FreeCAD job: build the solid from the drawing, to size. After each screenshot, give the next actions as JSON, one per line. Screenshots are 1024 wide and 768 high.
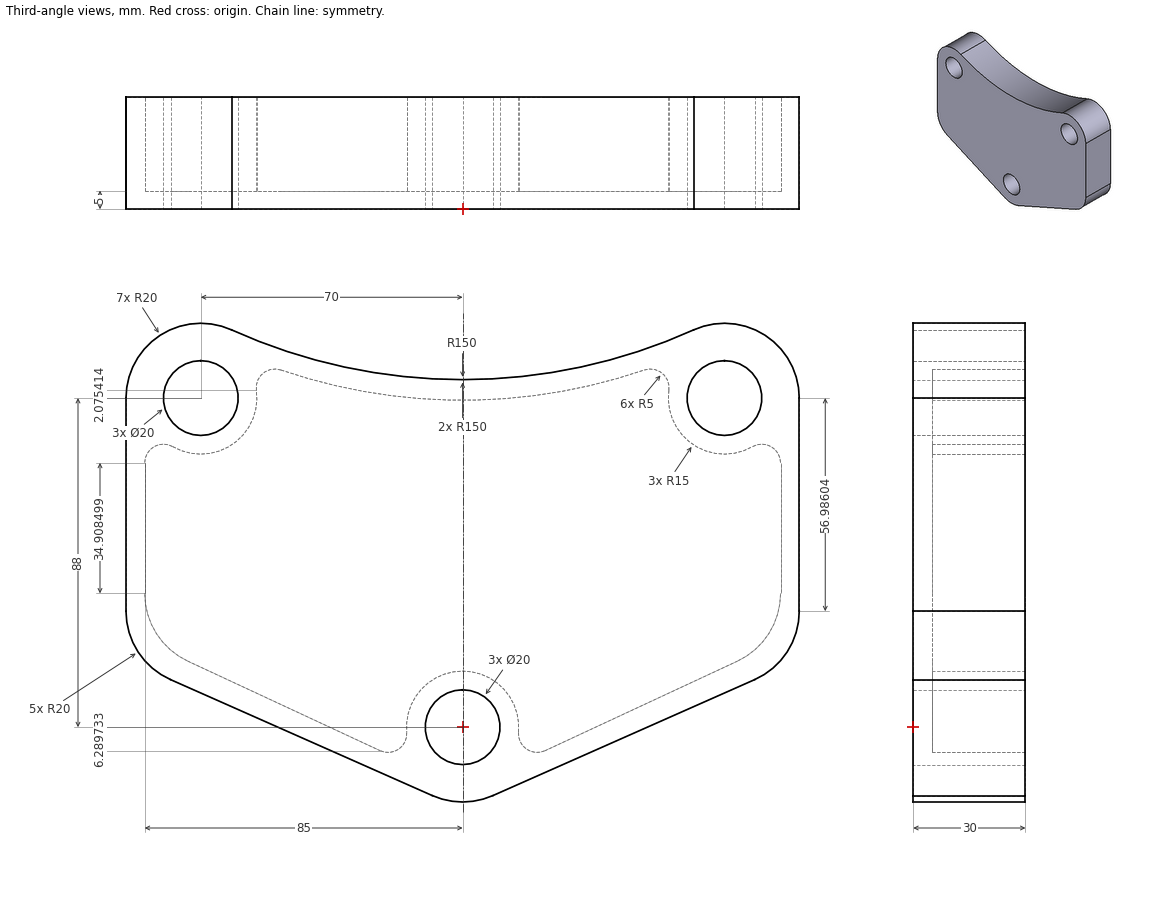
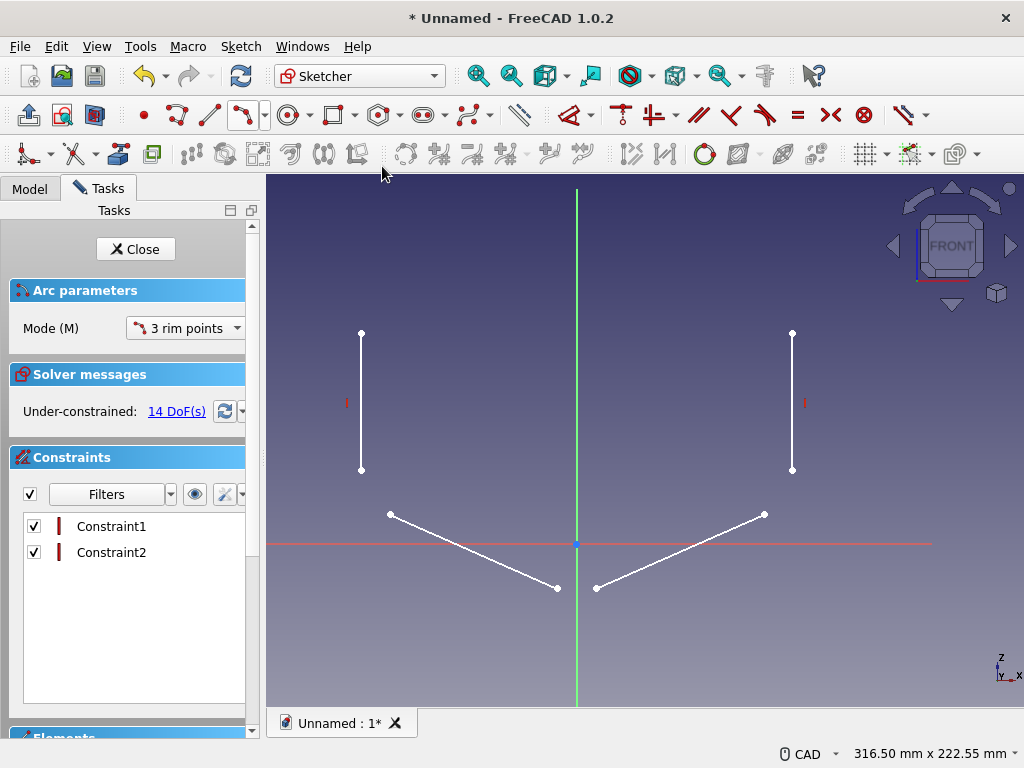
{"action": "left_click", "coordinate": [792, 471]}
{"action": "left_click", "coordinate": [764, 515]}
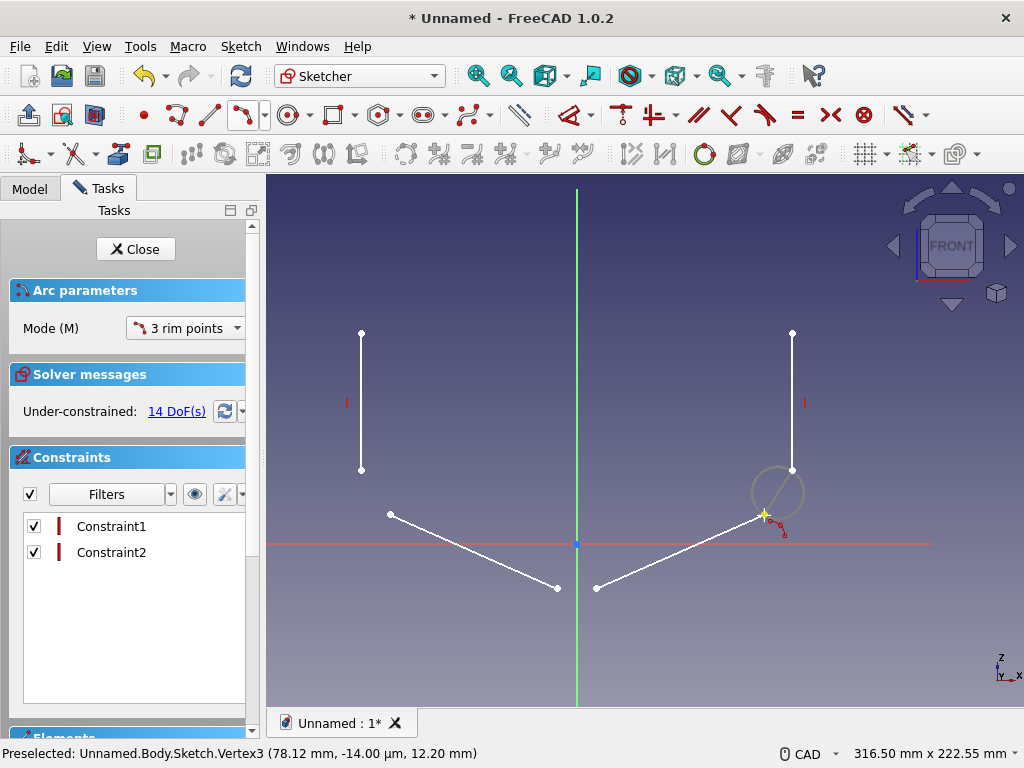
{"action": "scroll", "coordinate": [785, 496], "scroll_direction": "up", "scroll_amount": 4}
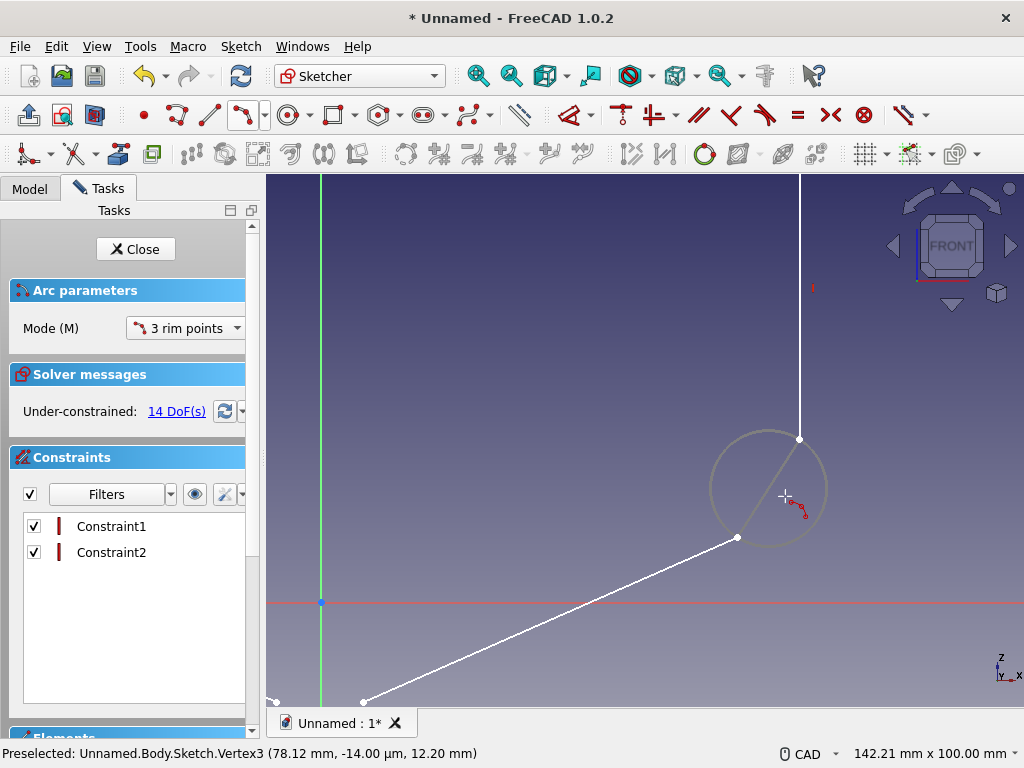
{"action": "left_click", "coordinate": [783, 495]}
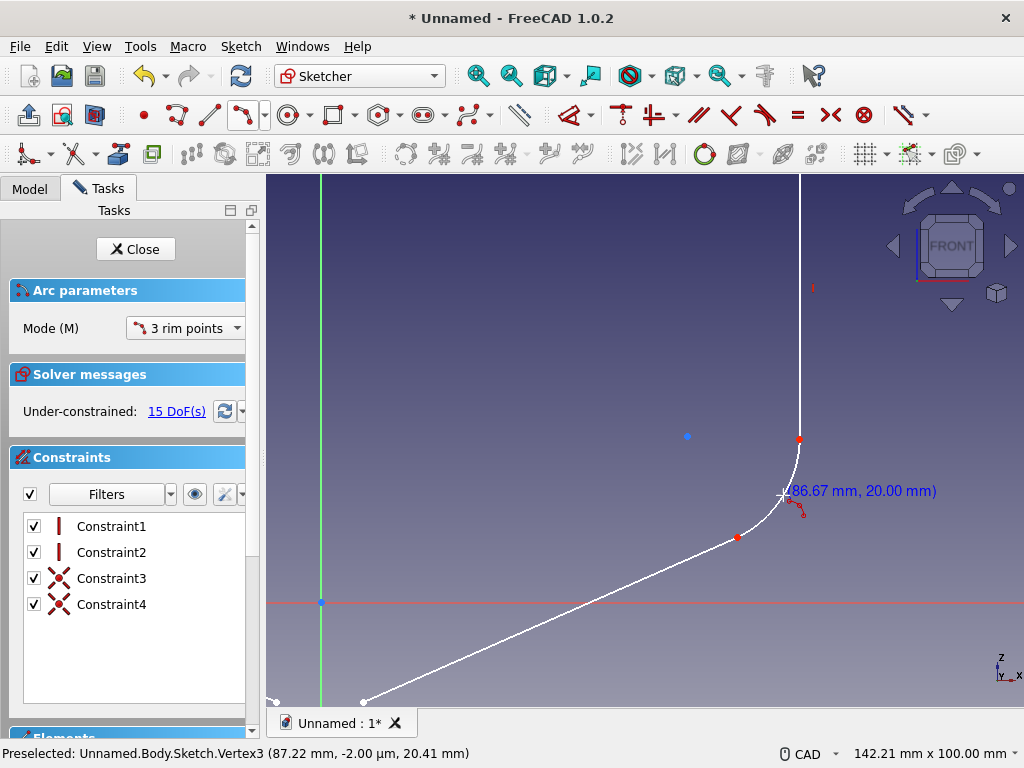
{"action": "scroll", "coordinate": [785, 496], "scroll_direction": "down", "scroll_amount": 4}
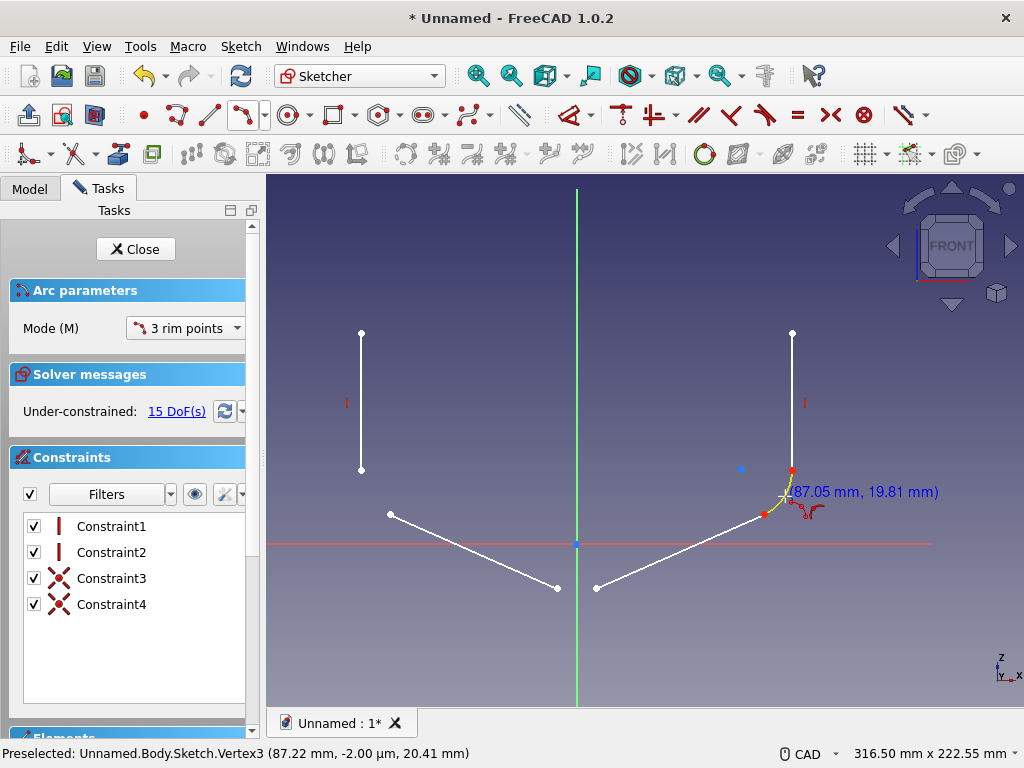
{"action": "left_click", "coordinate": [596, 589]}
{"action": "left_click", "coordinate": [557, 589]}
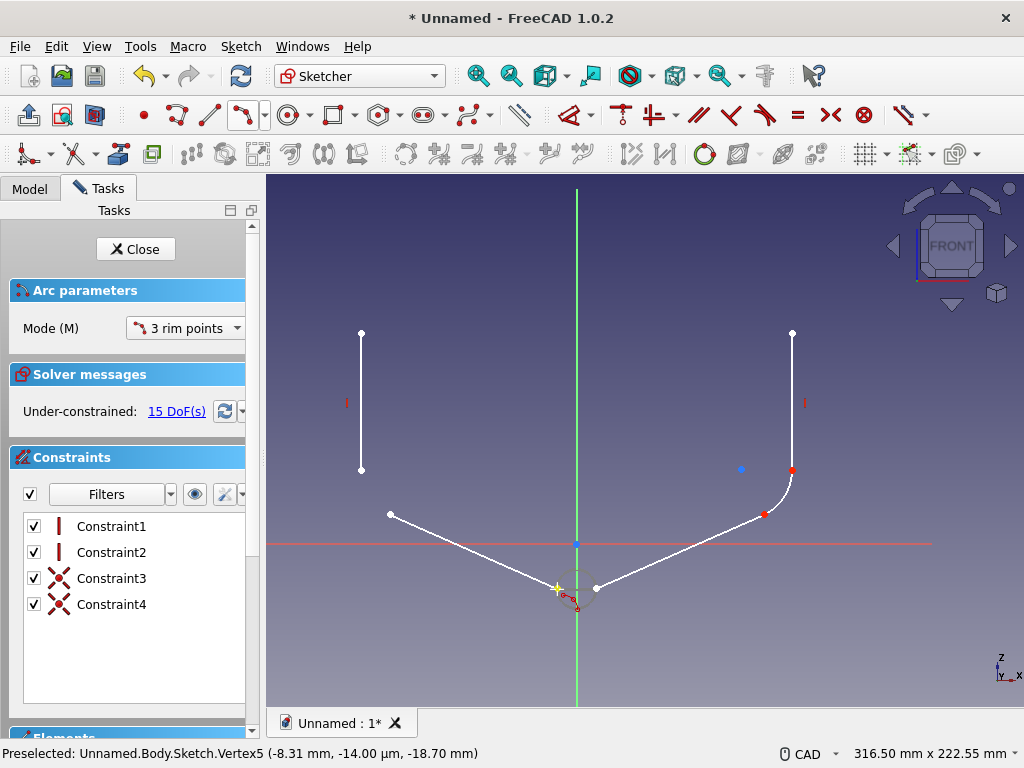
{"action": "scroll", "coordinate": [573, 592], "scroll_direction": "up", "scroll_amount": 7}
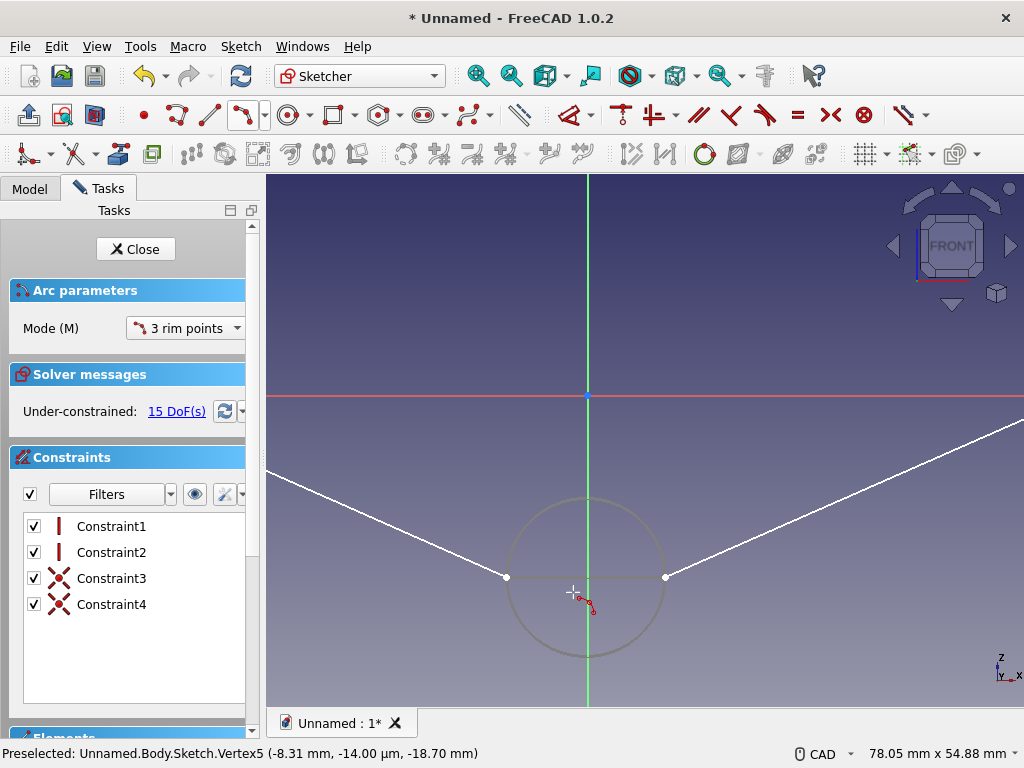
{"action": "left_click", "coordinate": [571, 589]}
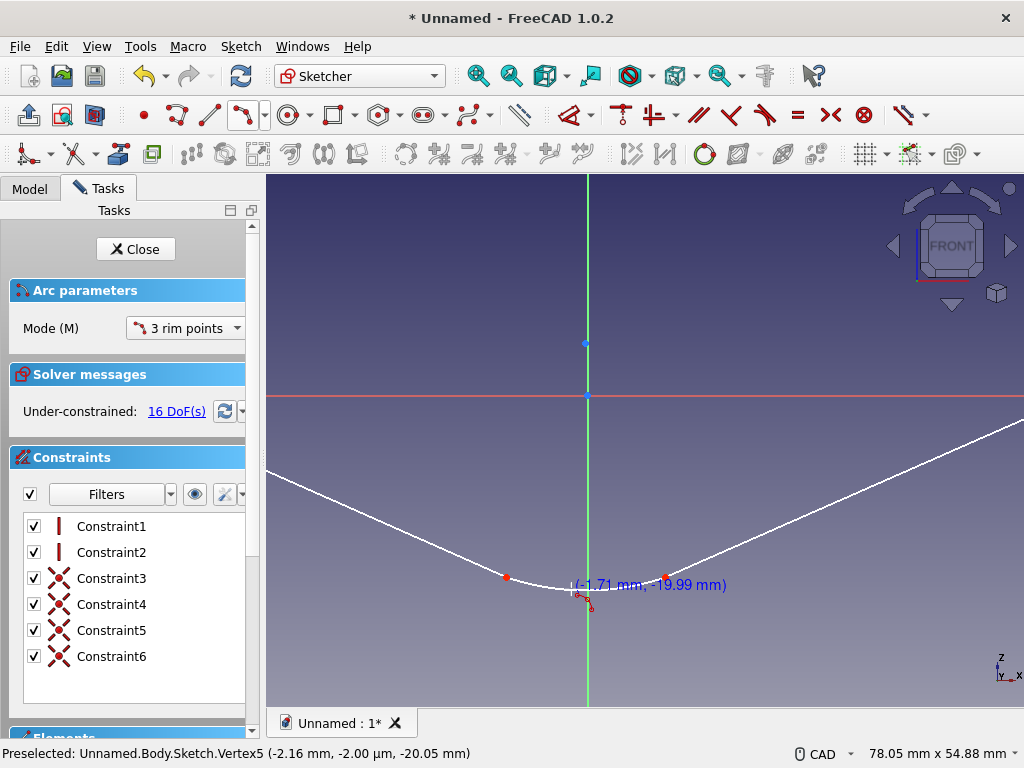
{"action": "scroll", "coordinate": [573, 592], "scroll_direction": "down", "scroll_amount": 7}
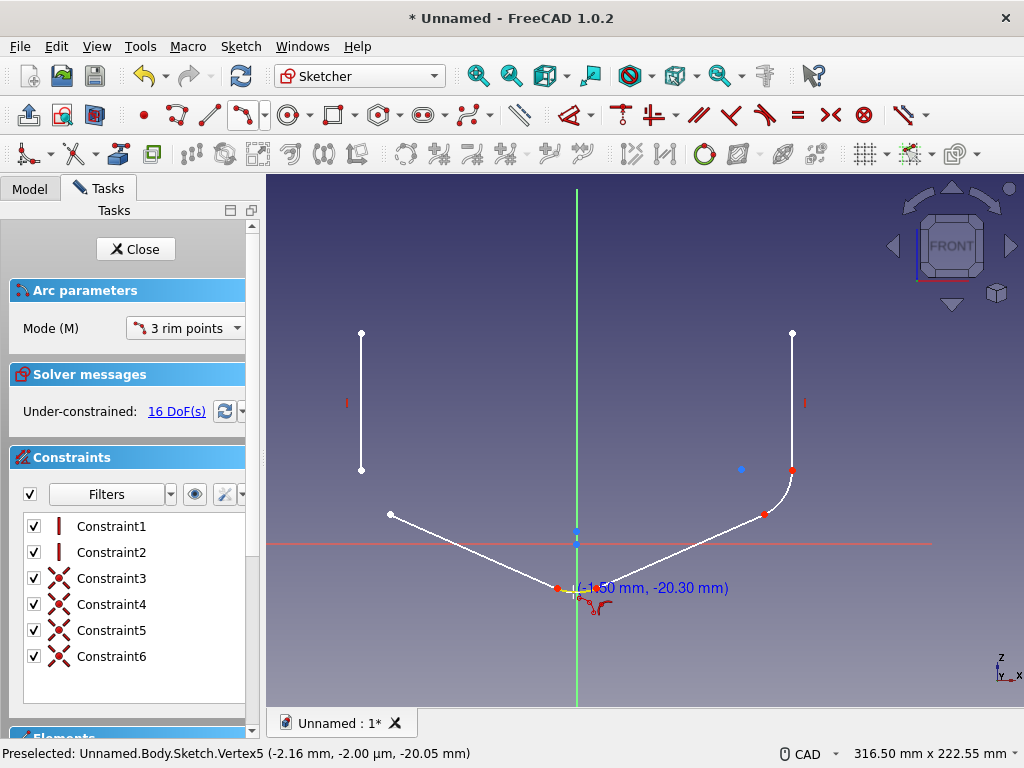
{"action": "left_click", "coordinate": [390, 515]}
{"action": "left_click", "coordinate": [361, 471]}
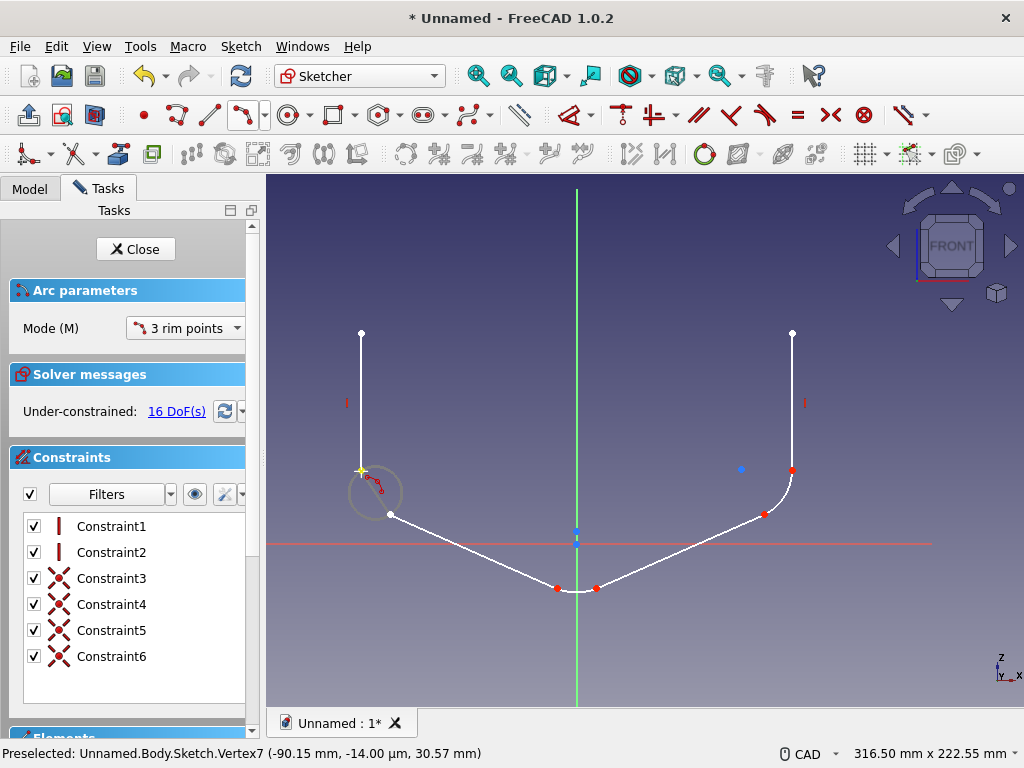
{"action": "scroll", "coordinate": [369, 496], "scroll_direction": "up", "scroll_amount": 4}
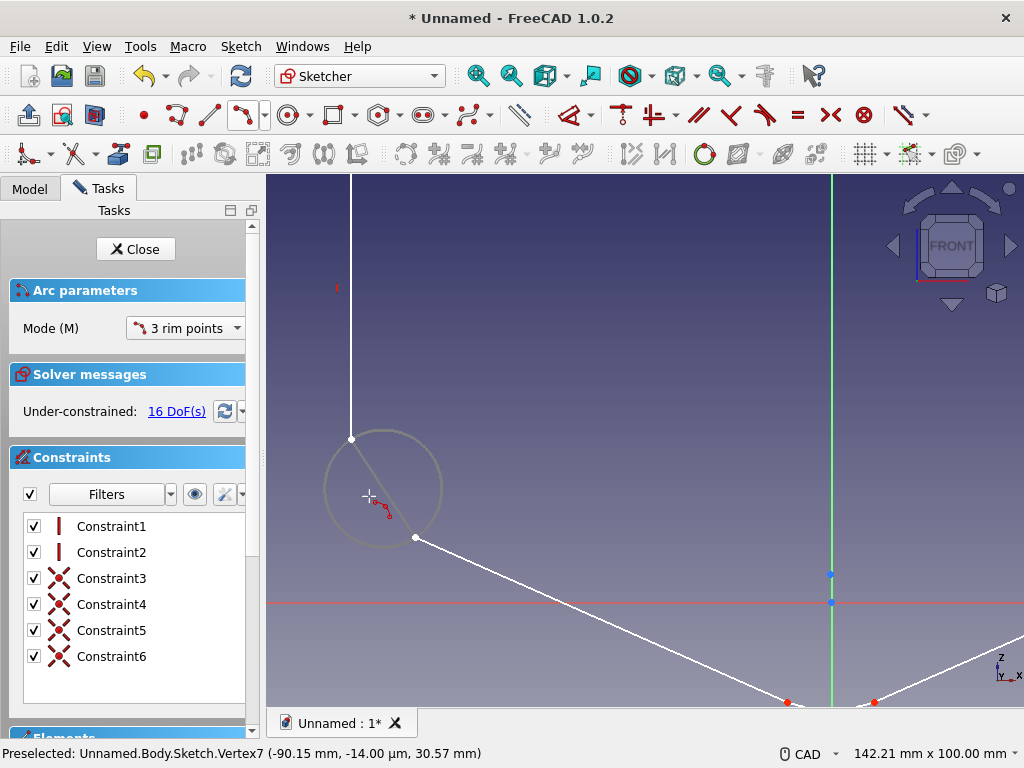
{"action": "left_click", "coordinate": [369, 495]}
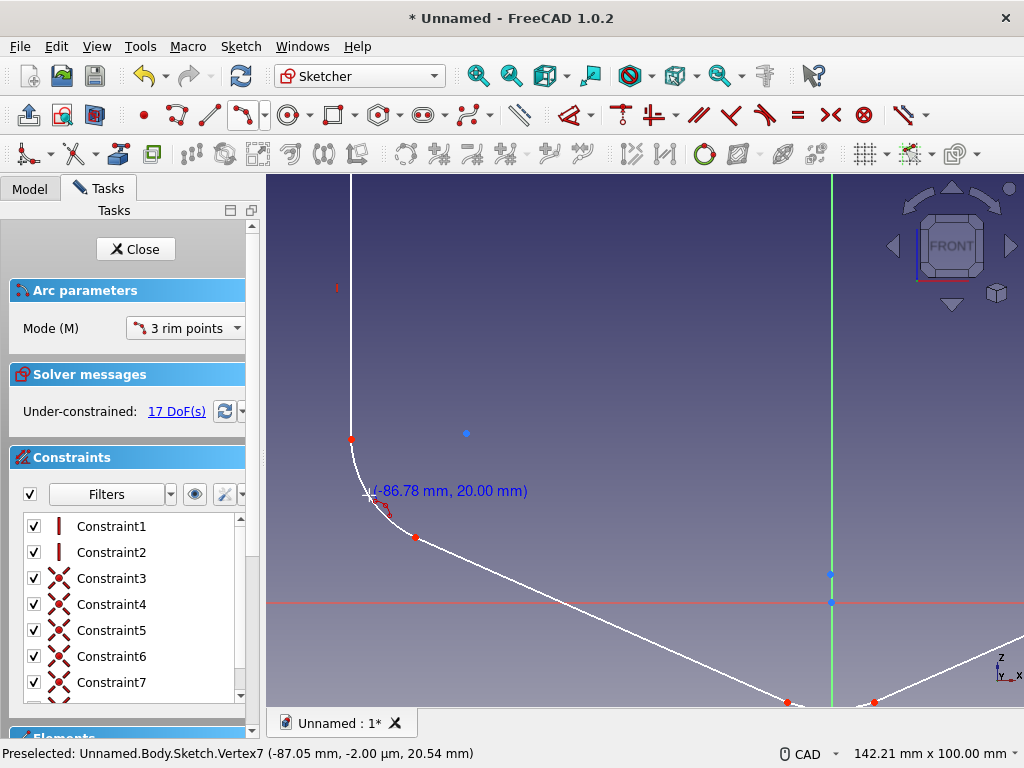
{"action": "scroll", "coordinate": [368, 496], "scroll_direction": "down", "scroll_amount": 4}